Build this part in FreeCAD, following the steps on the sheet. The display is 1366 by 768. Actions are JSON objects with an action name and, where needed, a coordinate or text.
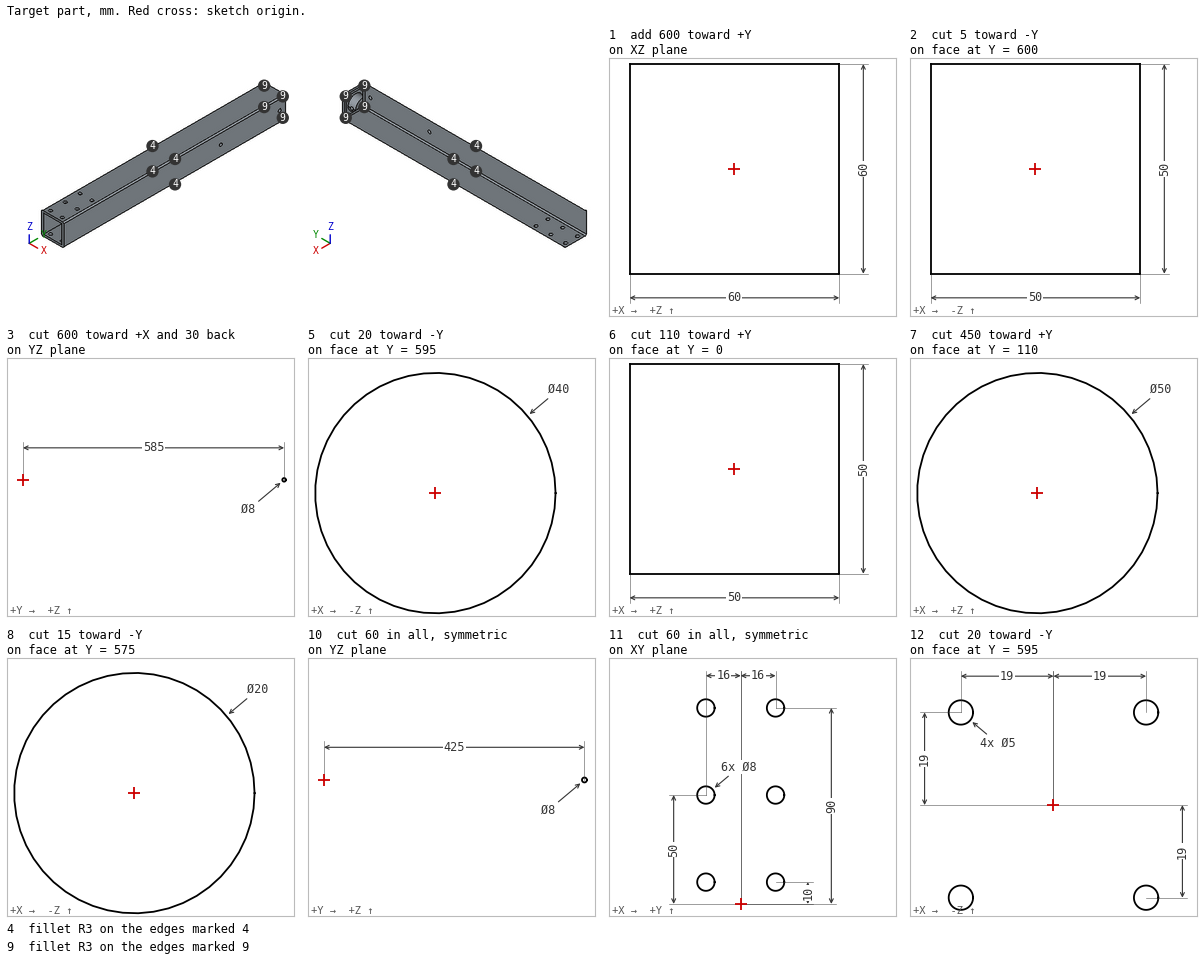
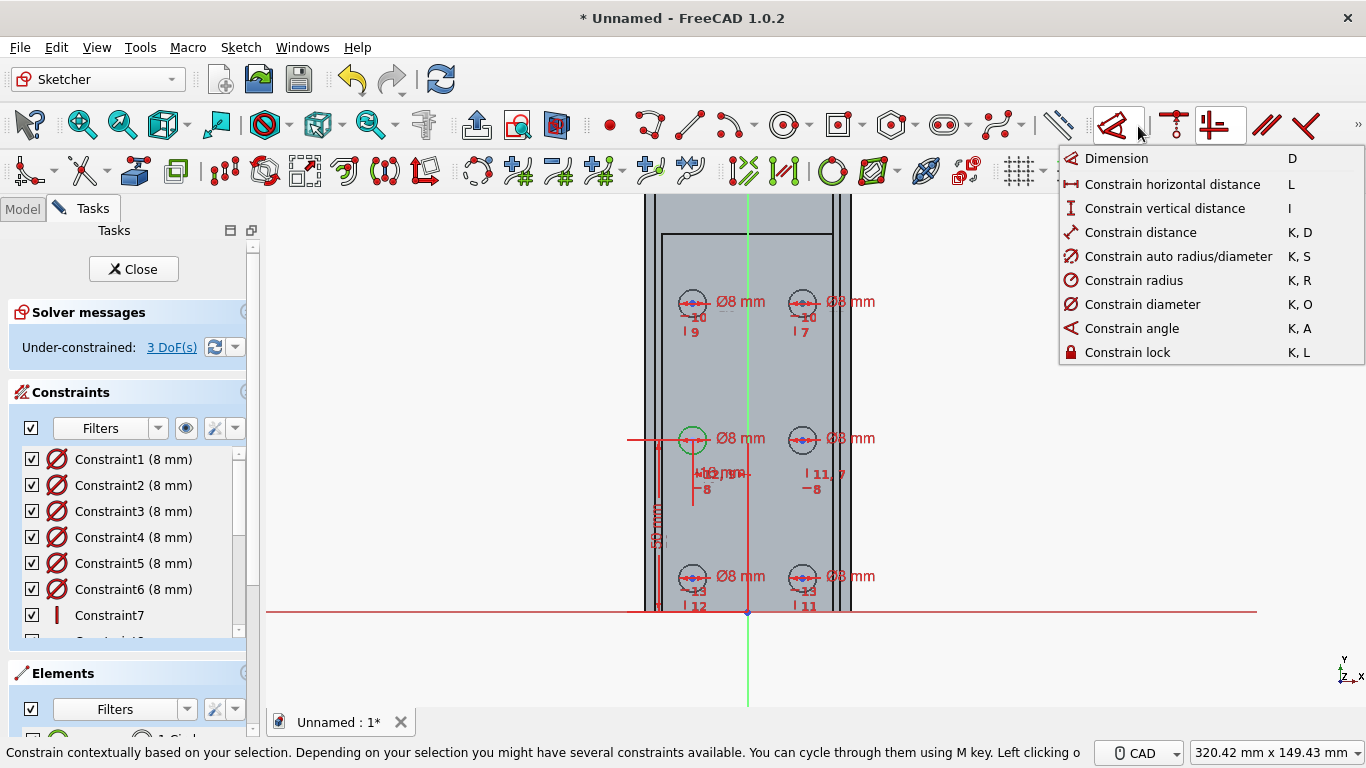
{"action": "left_click", "coordinate": [1212, 184]}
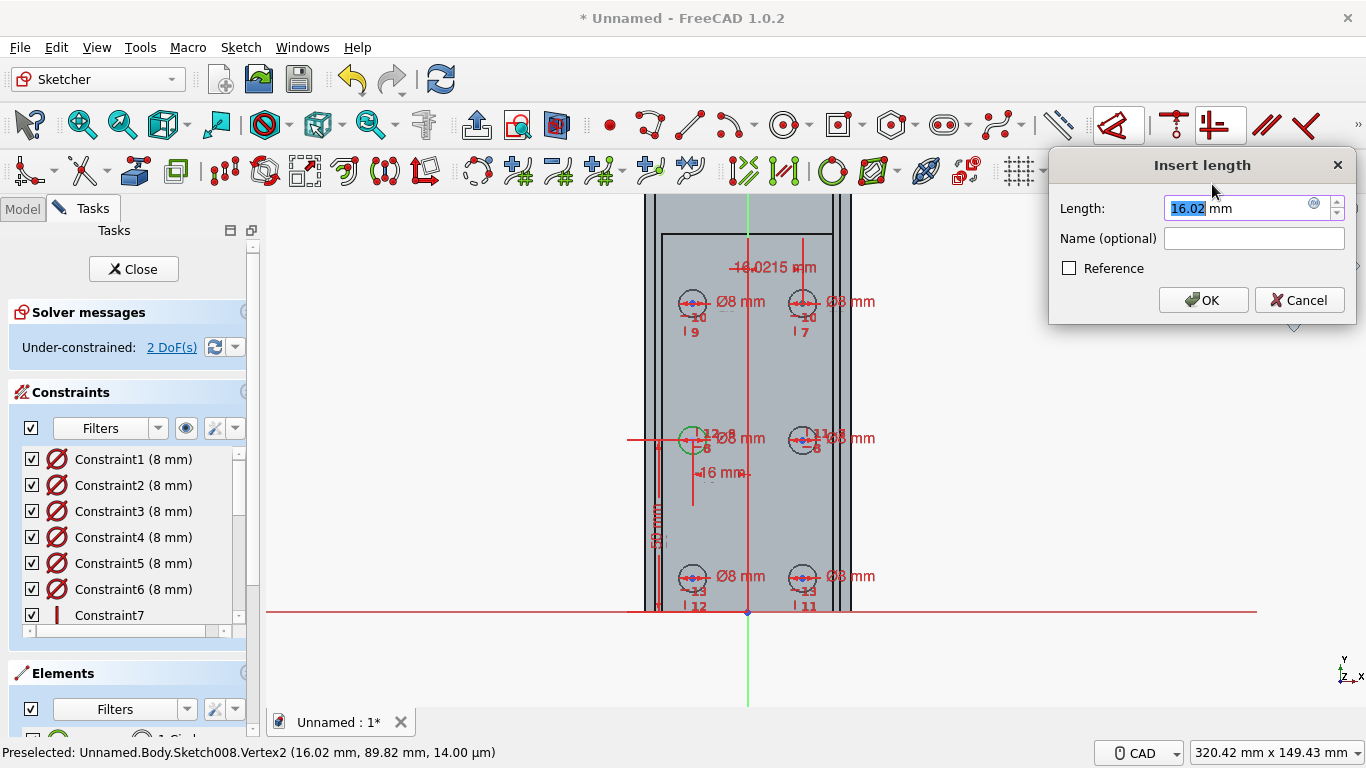
{"action": "type", "text": "16"}
{"action": "key", "text": "Return"}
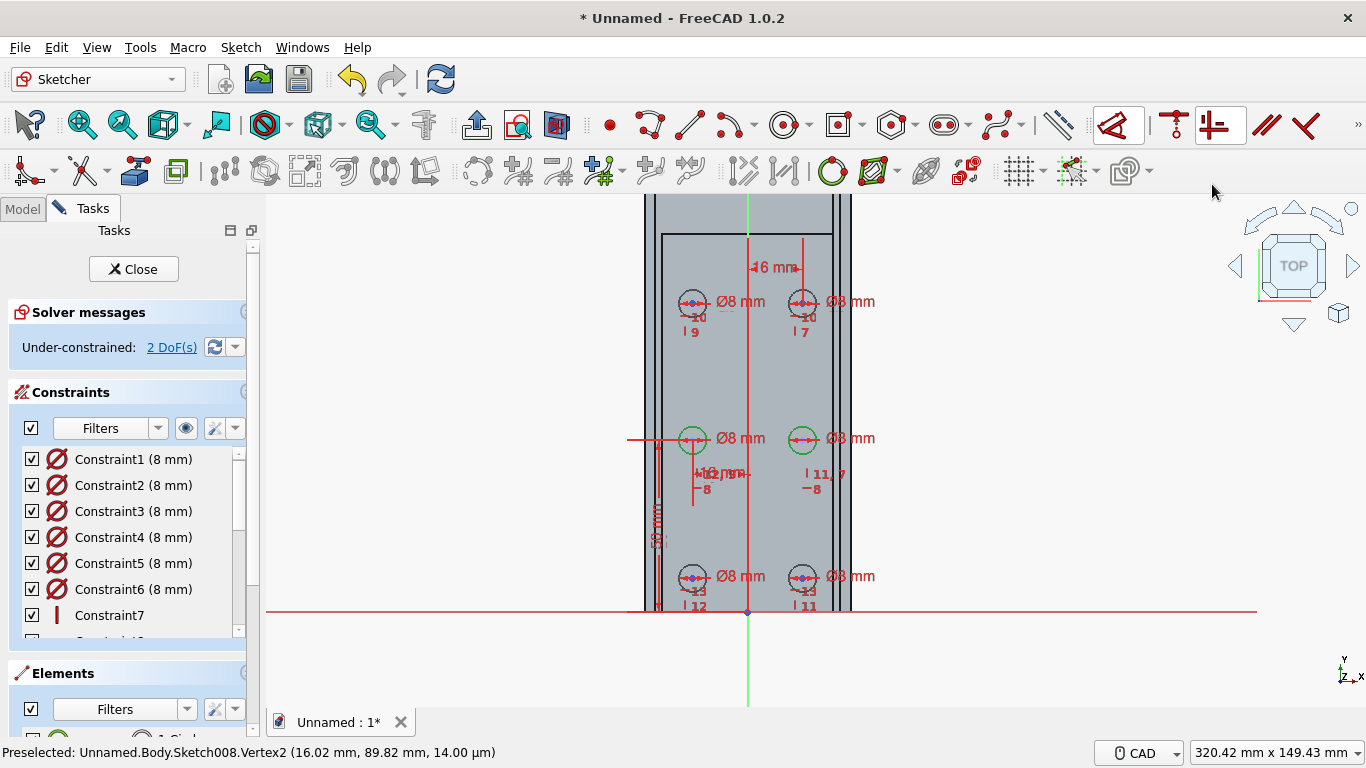
{"action": "left_click", "coordinate": [803, 304]}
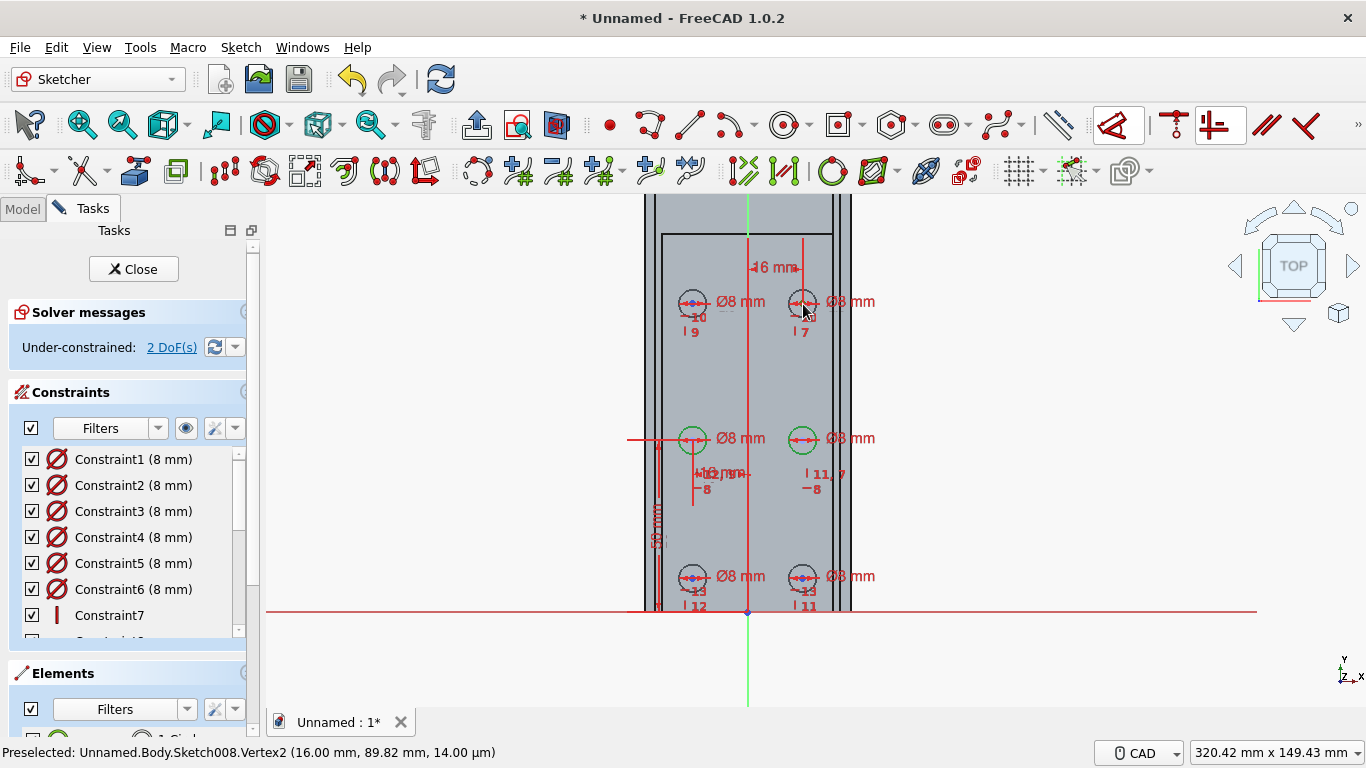
{"action": "key", "text": "i"}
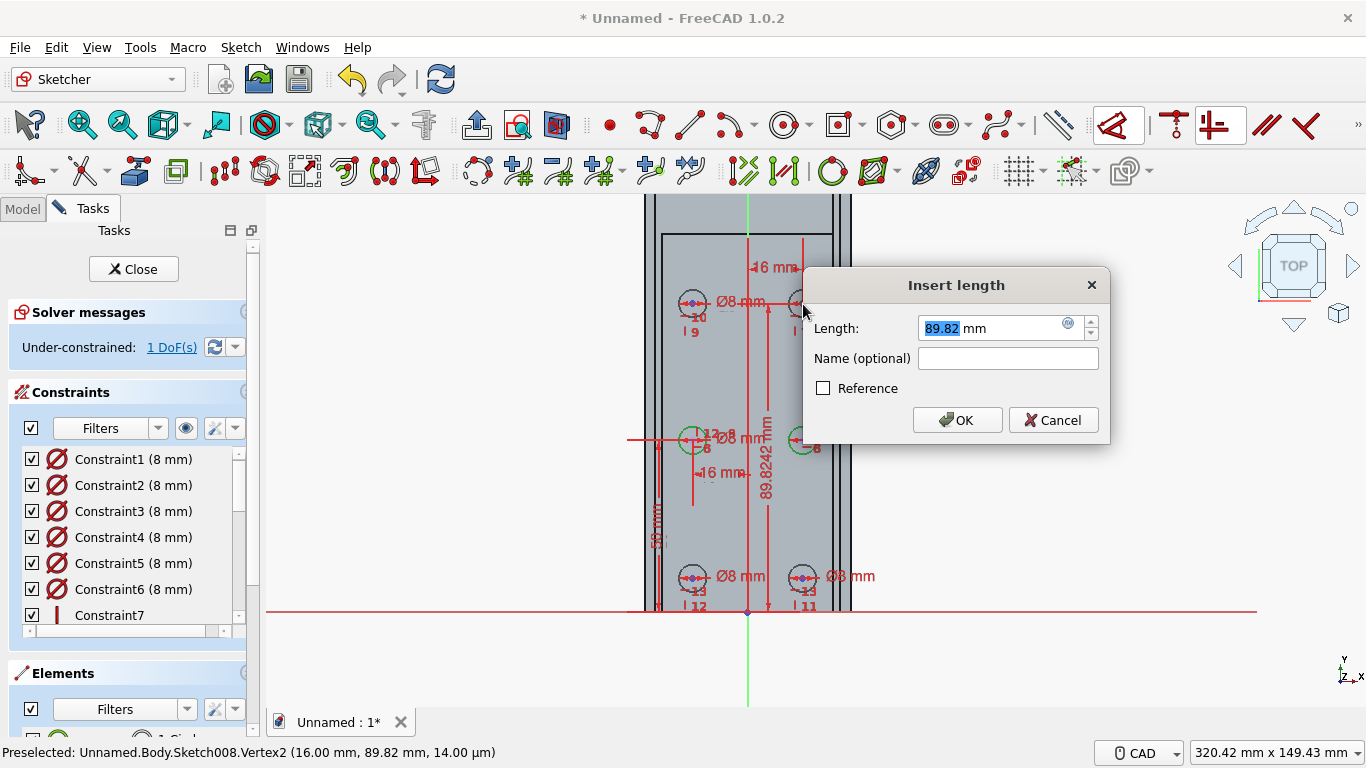
{"action": "type", "text": "90"}
{"action": "key", "text": "Return"}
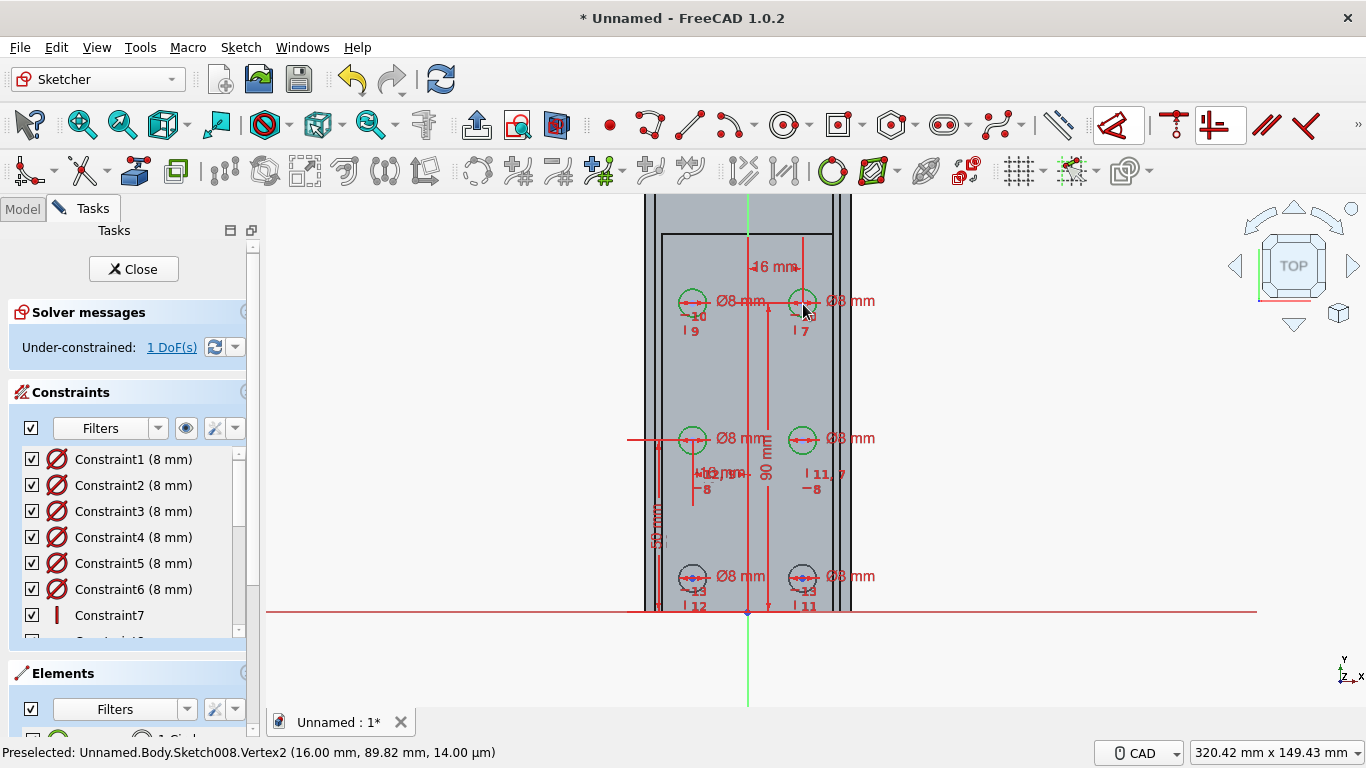
{"action": "left_click", "coordinate": [803, 578]}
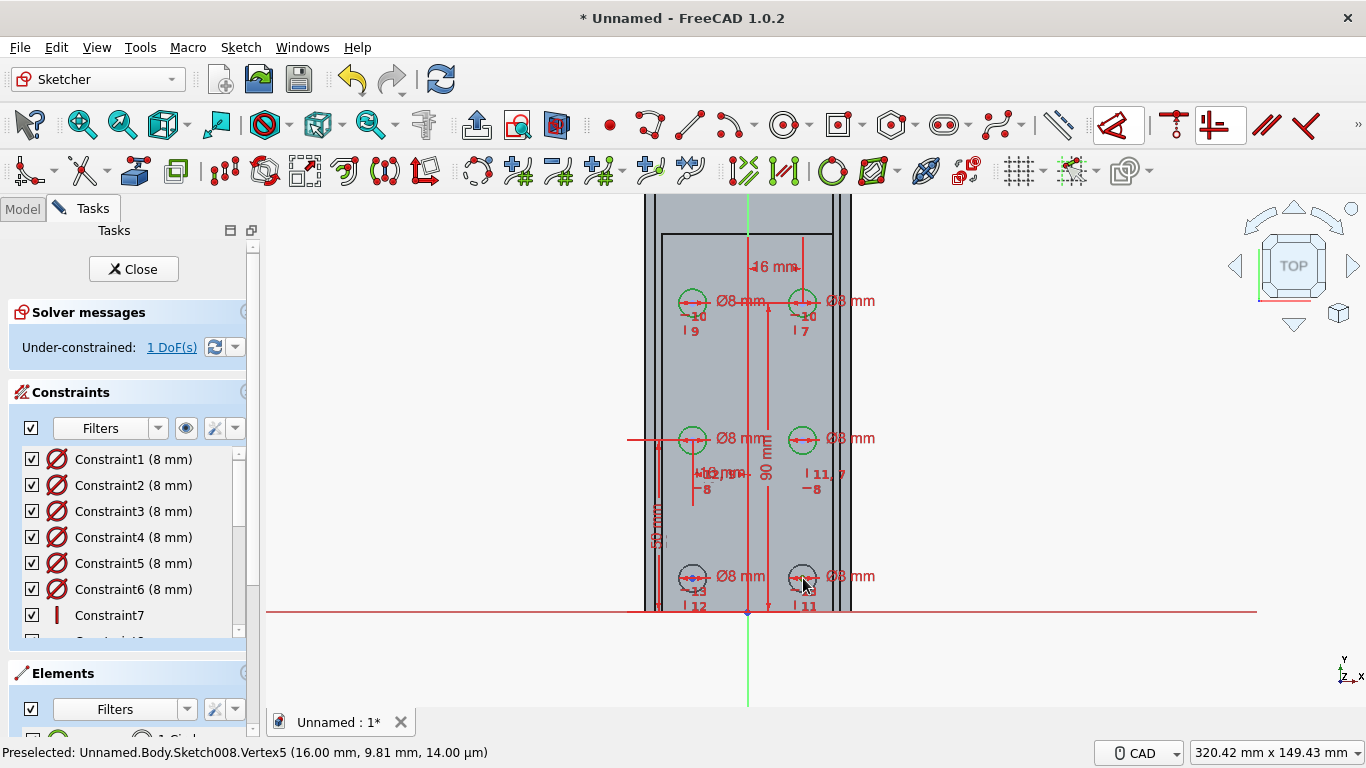
{"action": "key", "text": "i"}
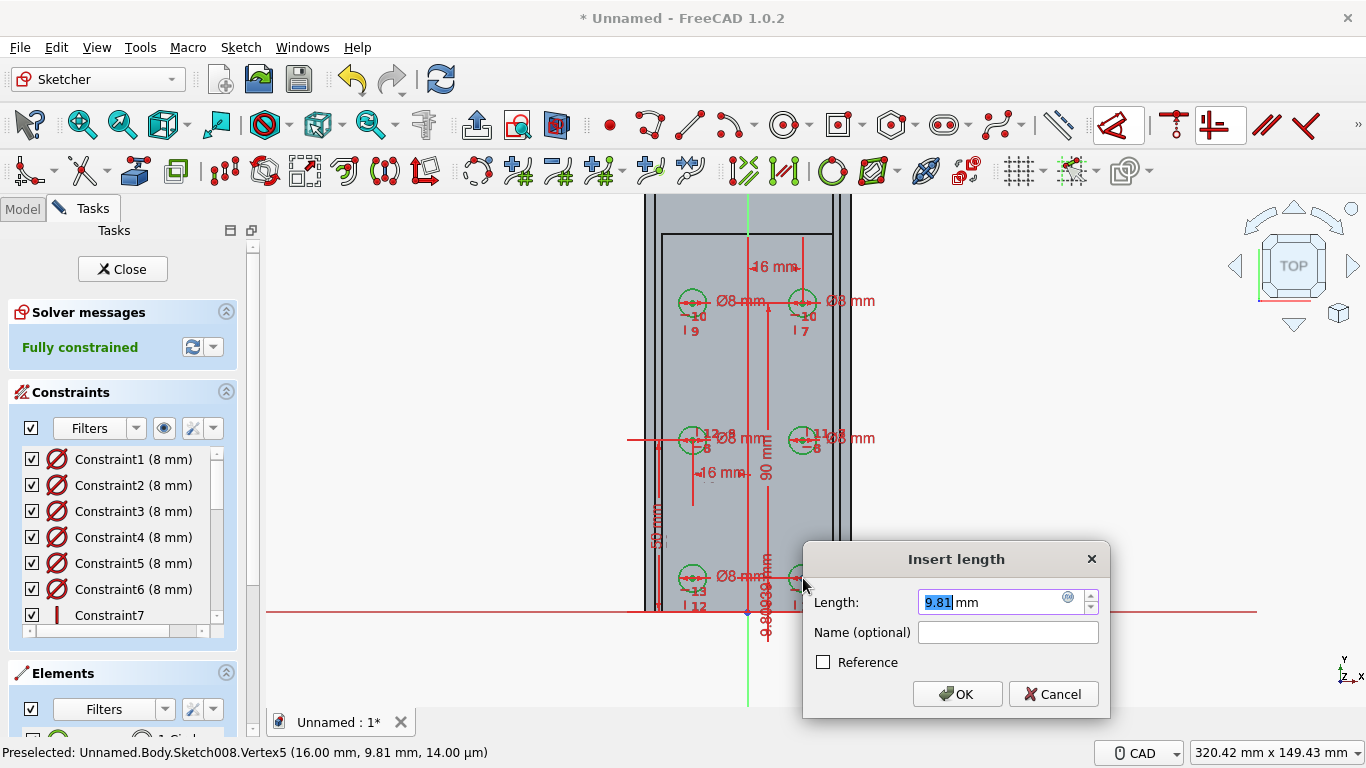
{"action": "type", "text": "10"}
{"action": "key", "text": "Return"}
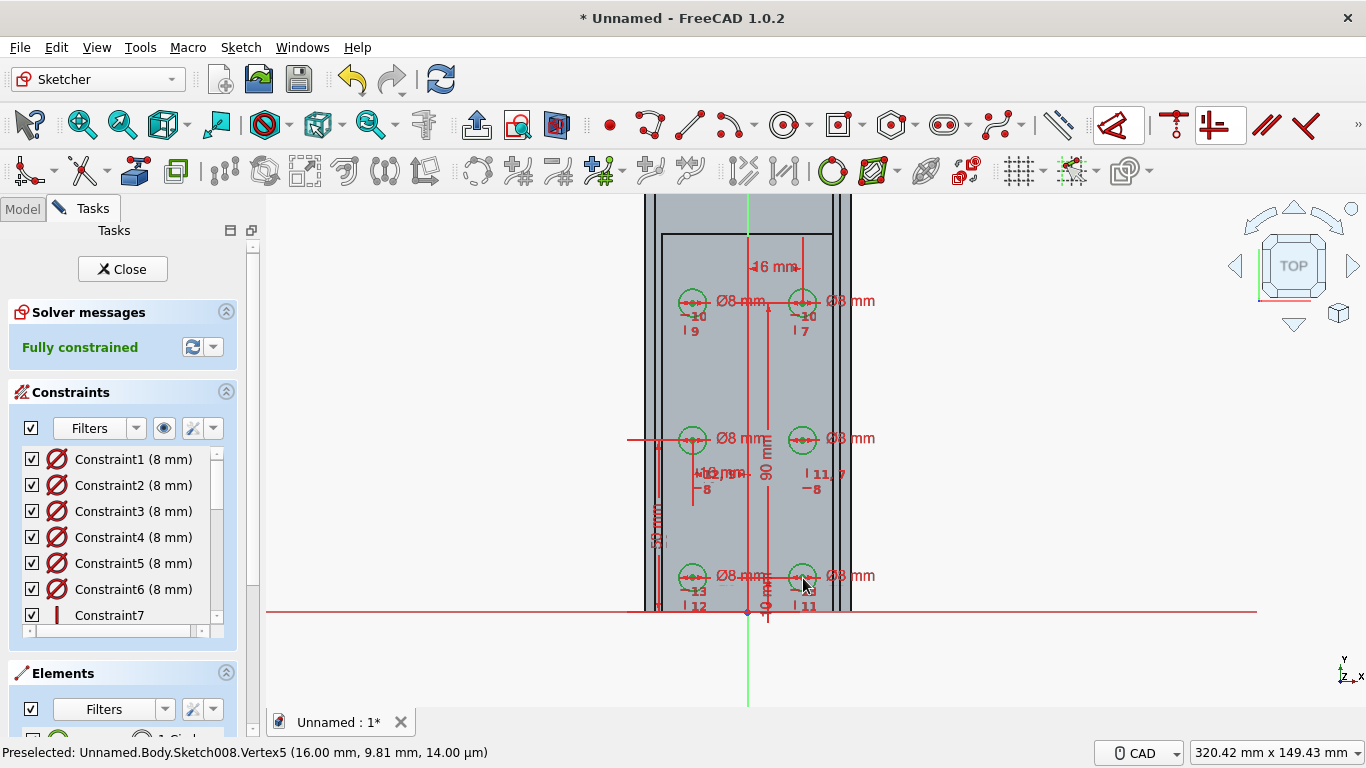
{"action": "left_click", "coordinate": [123, 269]}